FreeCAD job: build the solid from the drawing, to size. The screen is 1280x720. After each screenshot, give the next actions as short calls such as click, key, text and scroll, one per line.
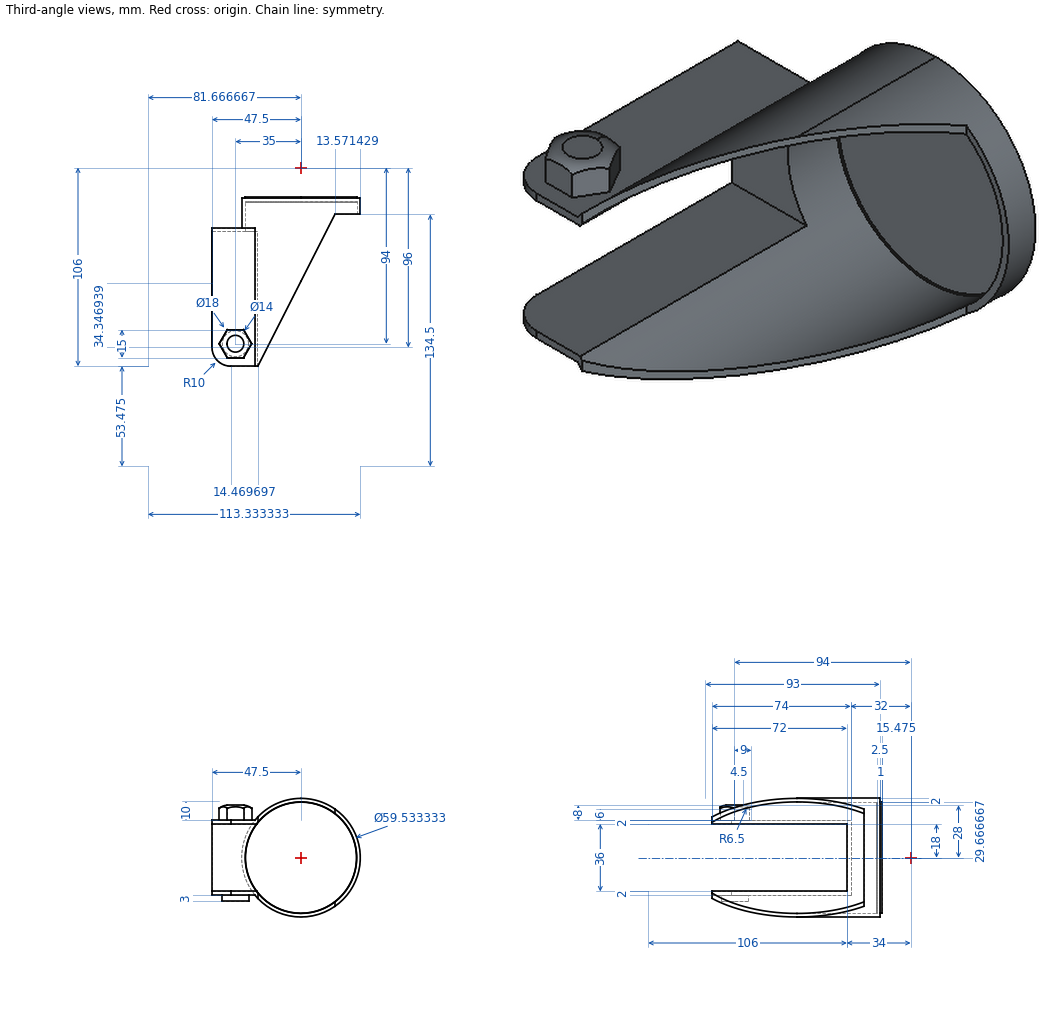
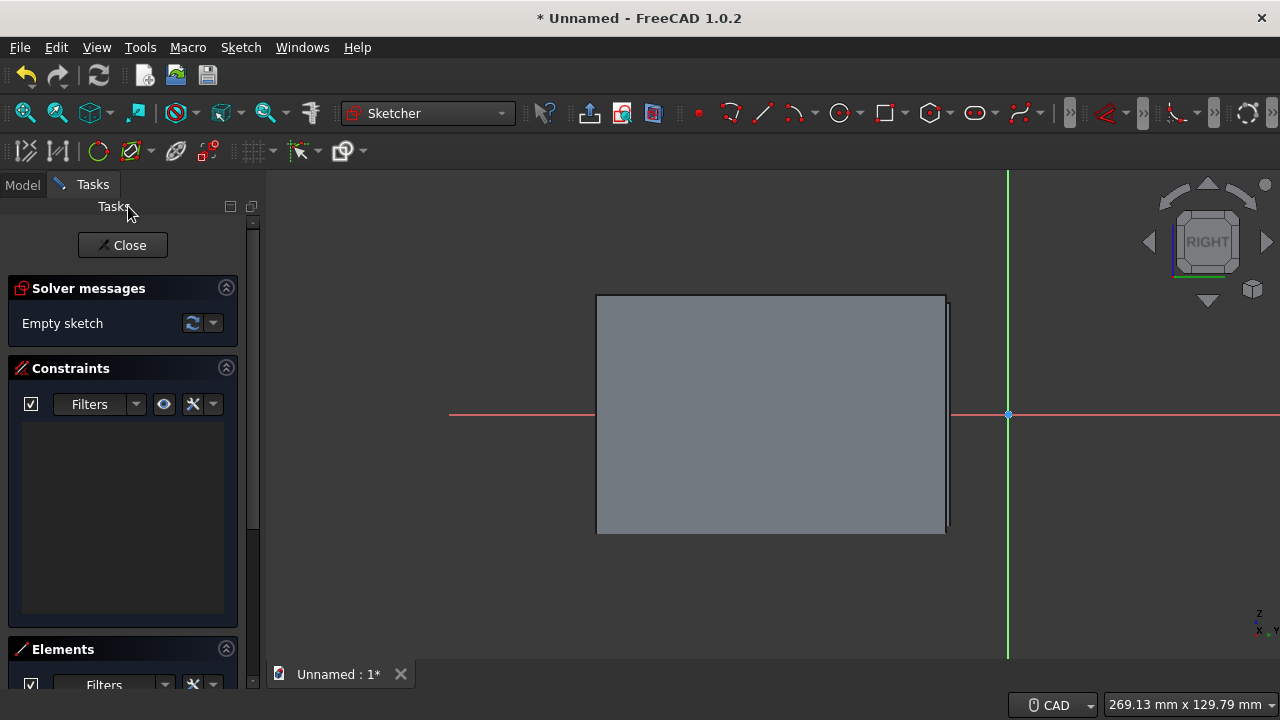
key(q)
key(s)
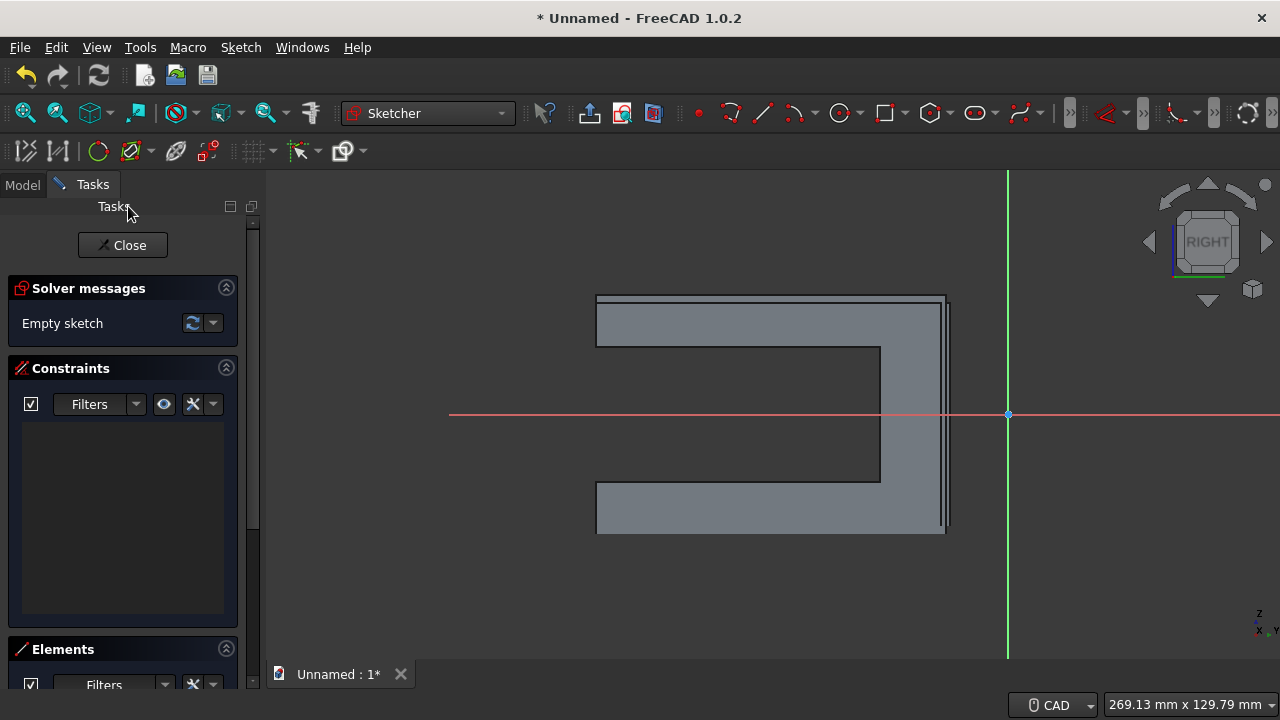
scroll(1021, 415, up, 2)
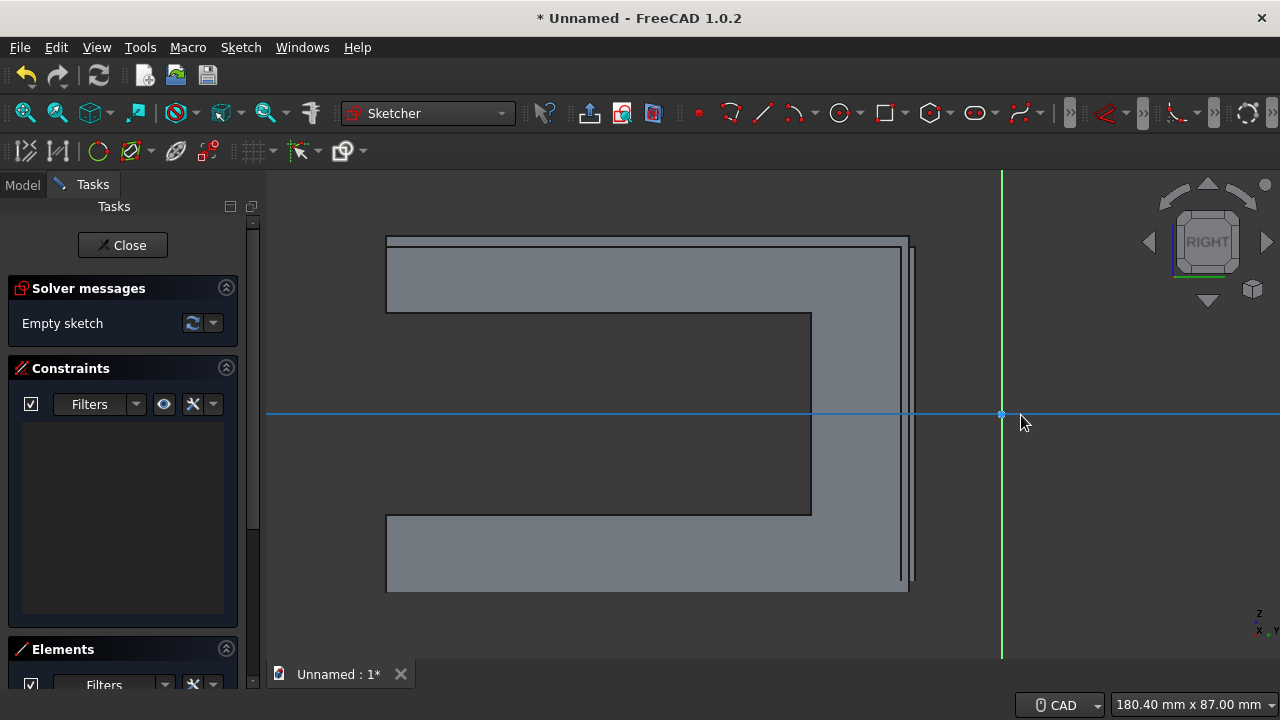
click(732, 114)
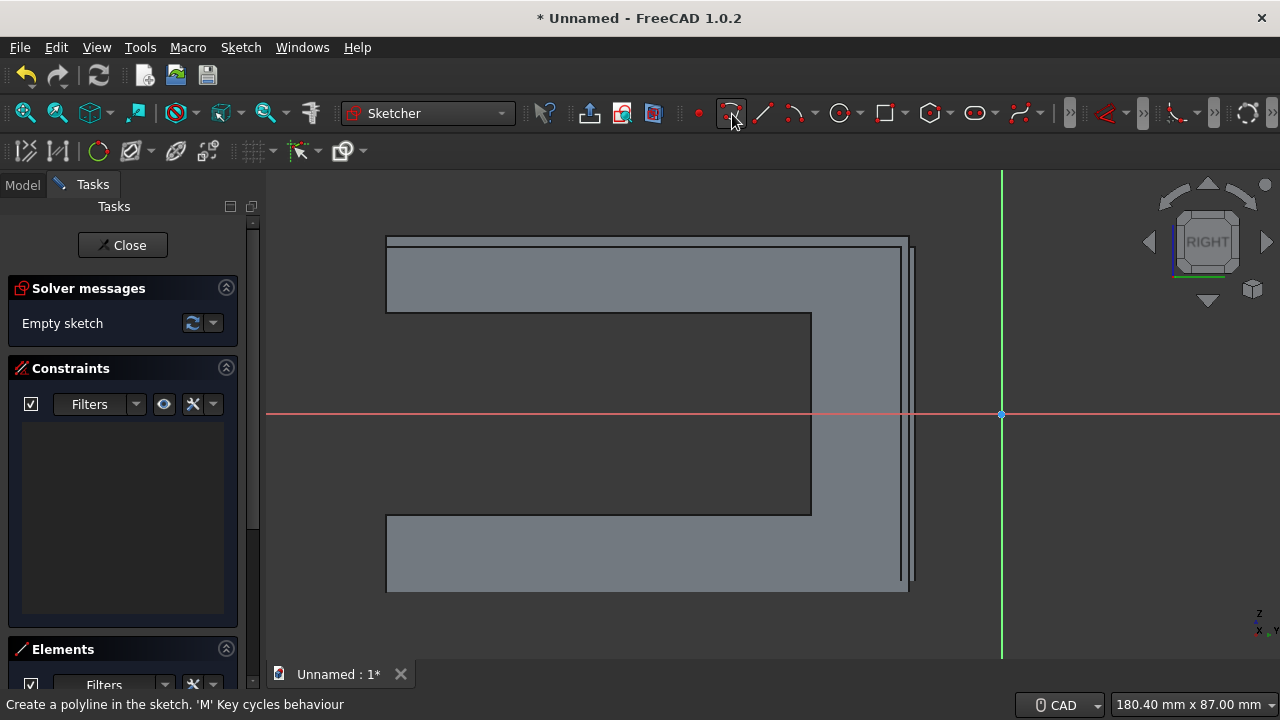
click(822, 302)
click(406, 302)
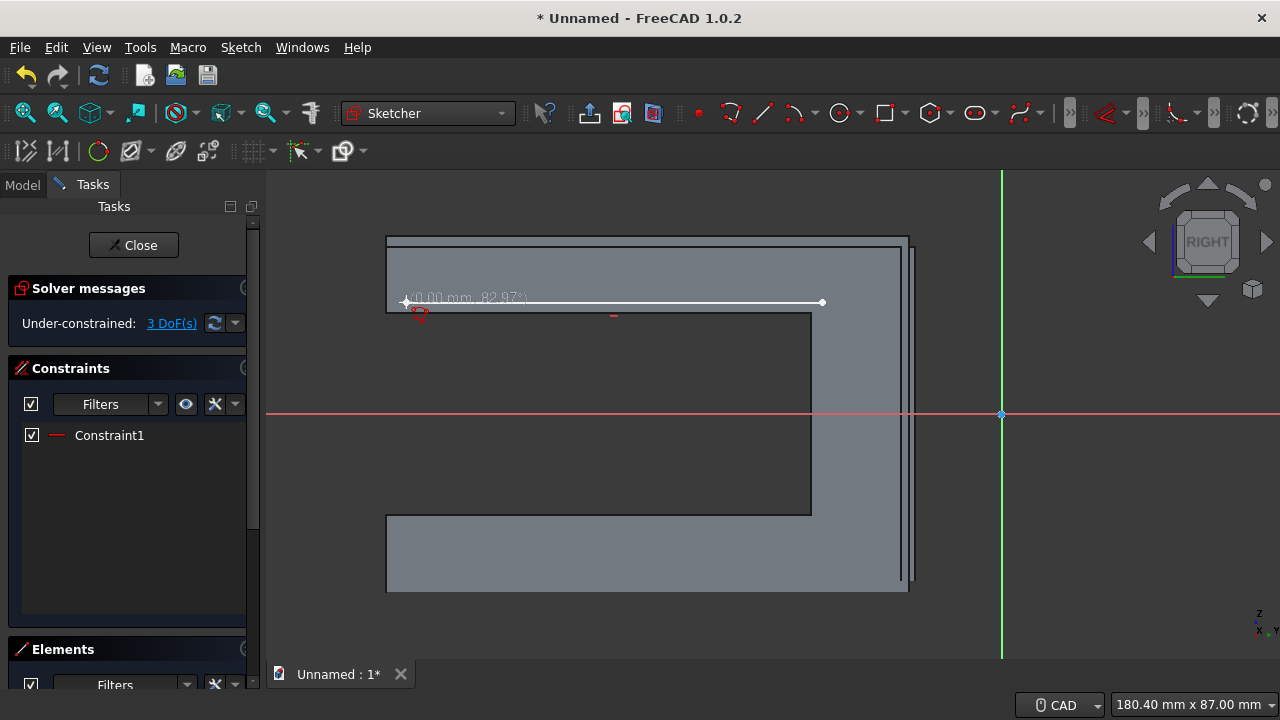
scroll(406, 313, up, 2)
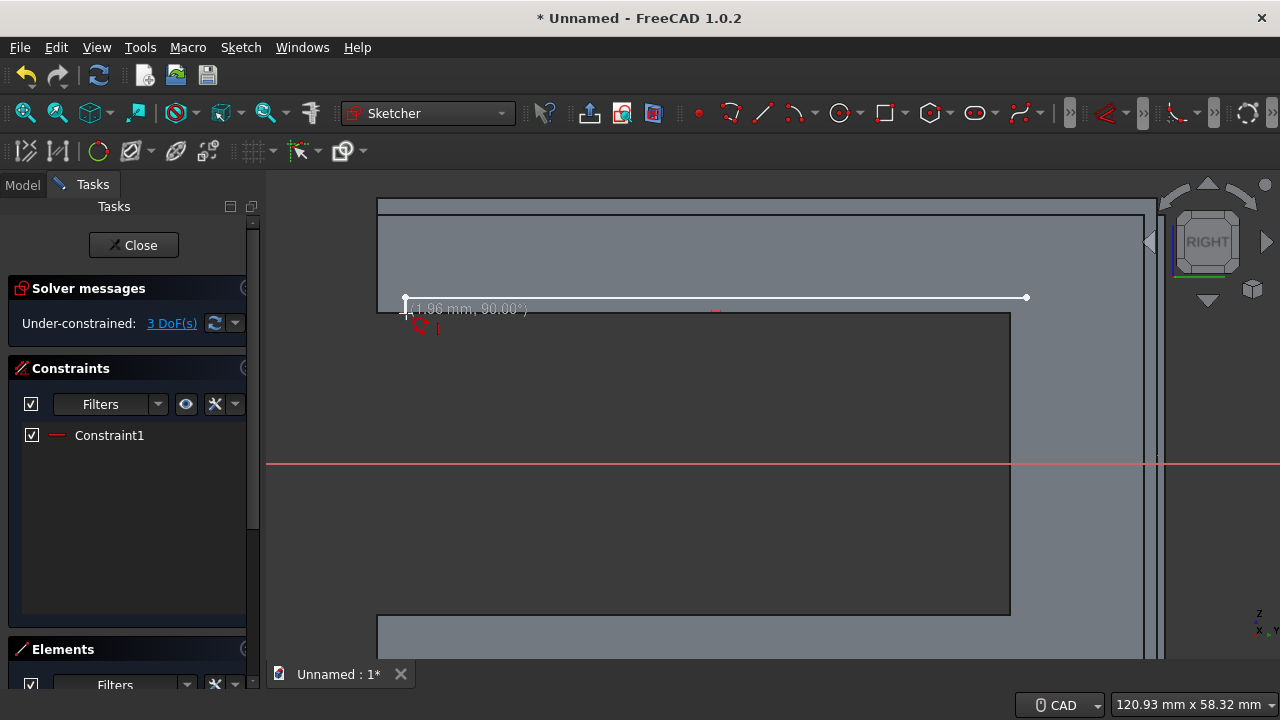
click(406, 313)
click(1010, 313)
click(1010, 615)
click(406, 615)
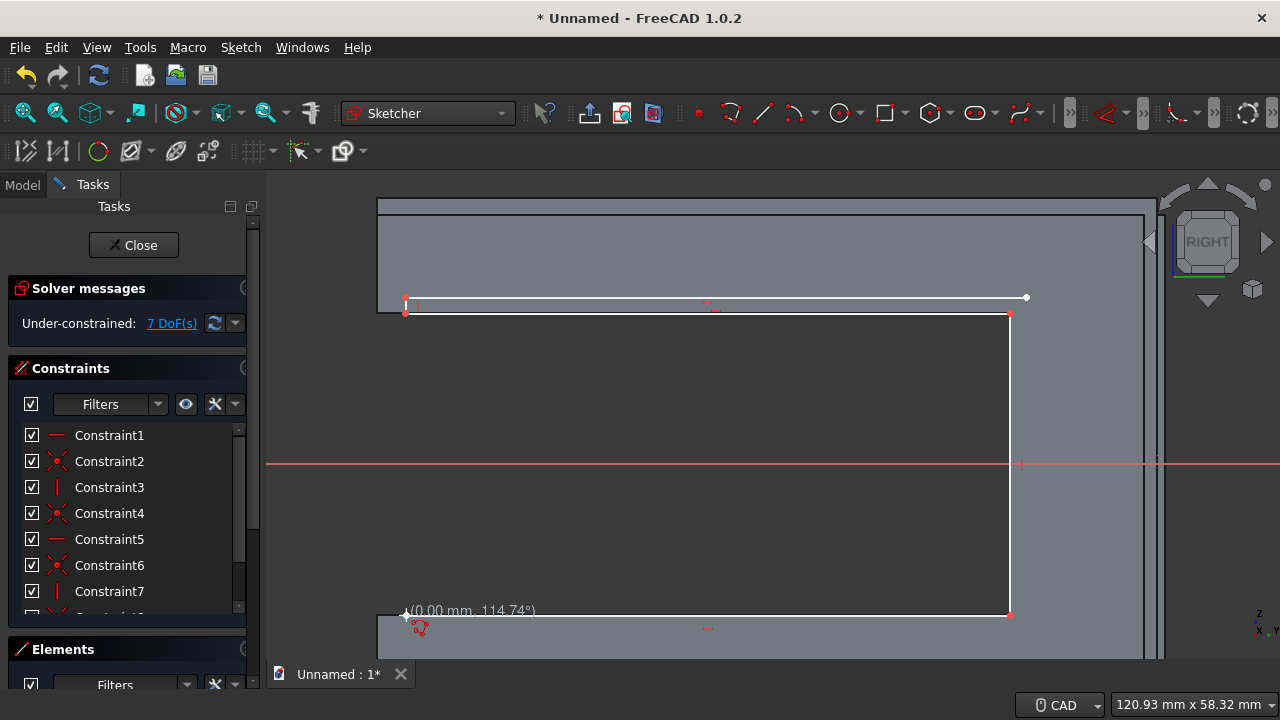
scroll(408, 314, down, 2)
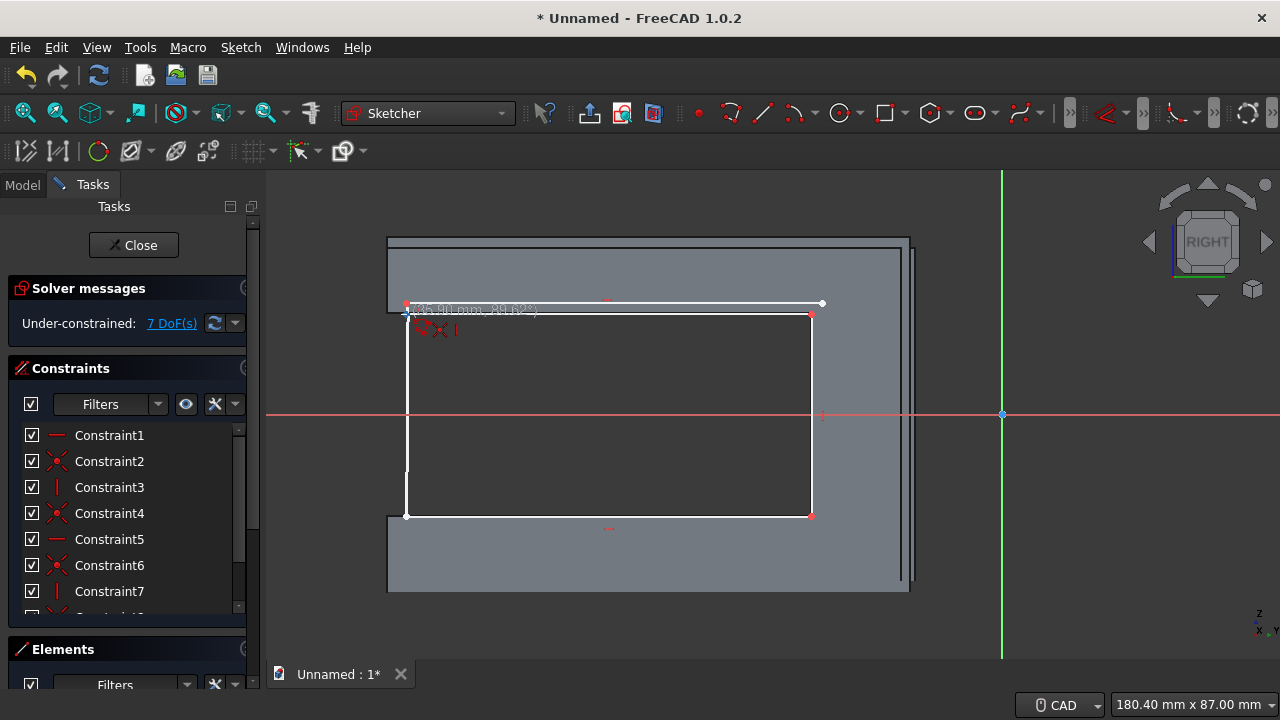
scroll(407, 527, up, 2)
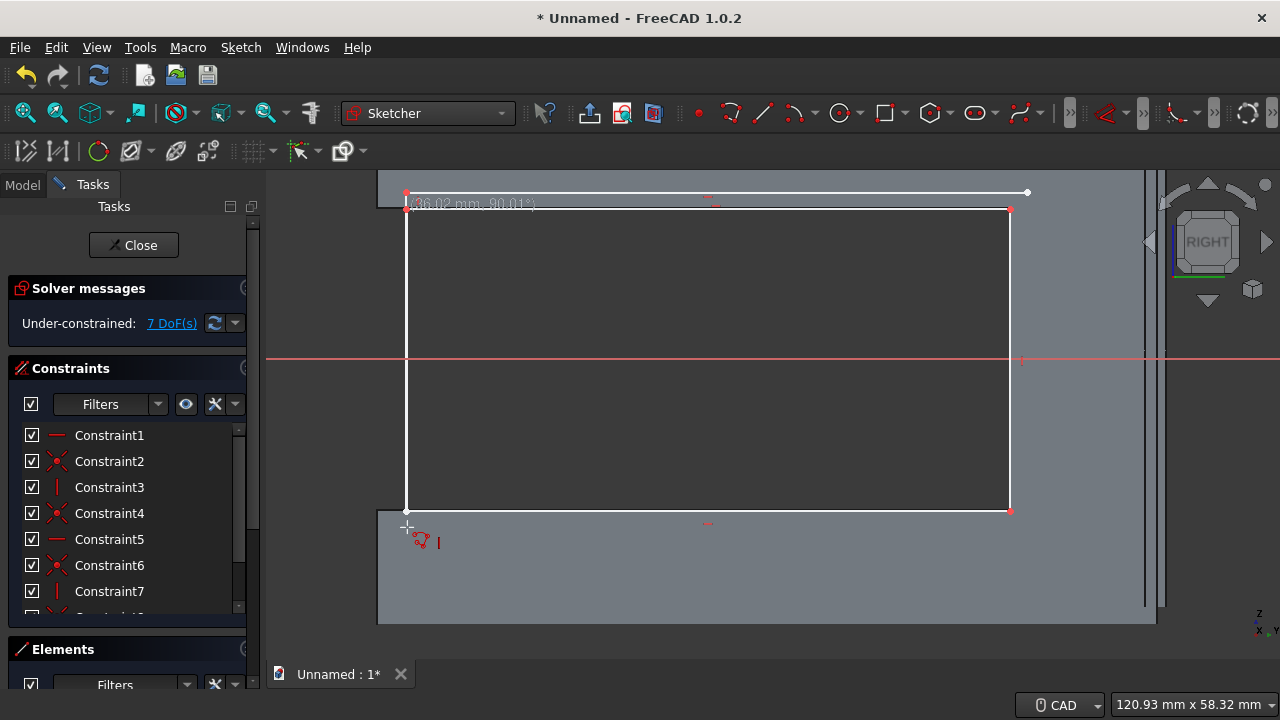
click(406, 527)
click(1027, 527)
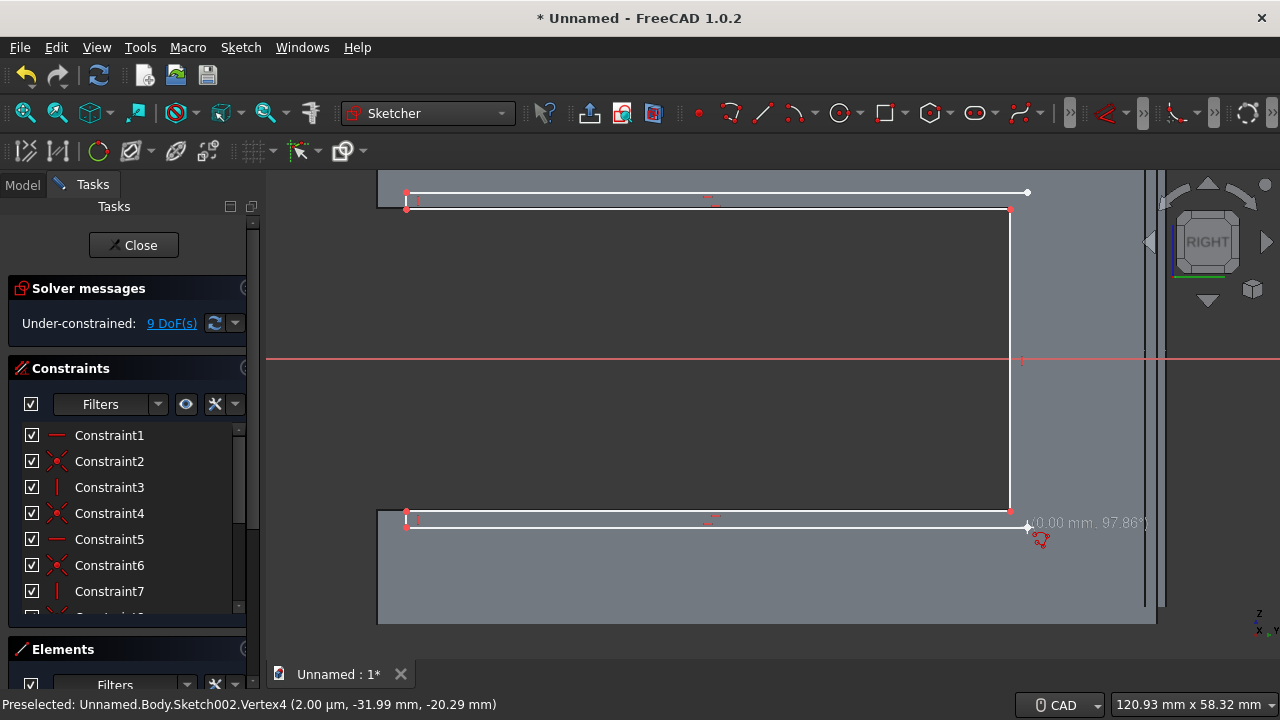
scroll(407, 528, down, 2)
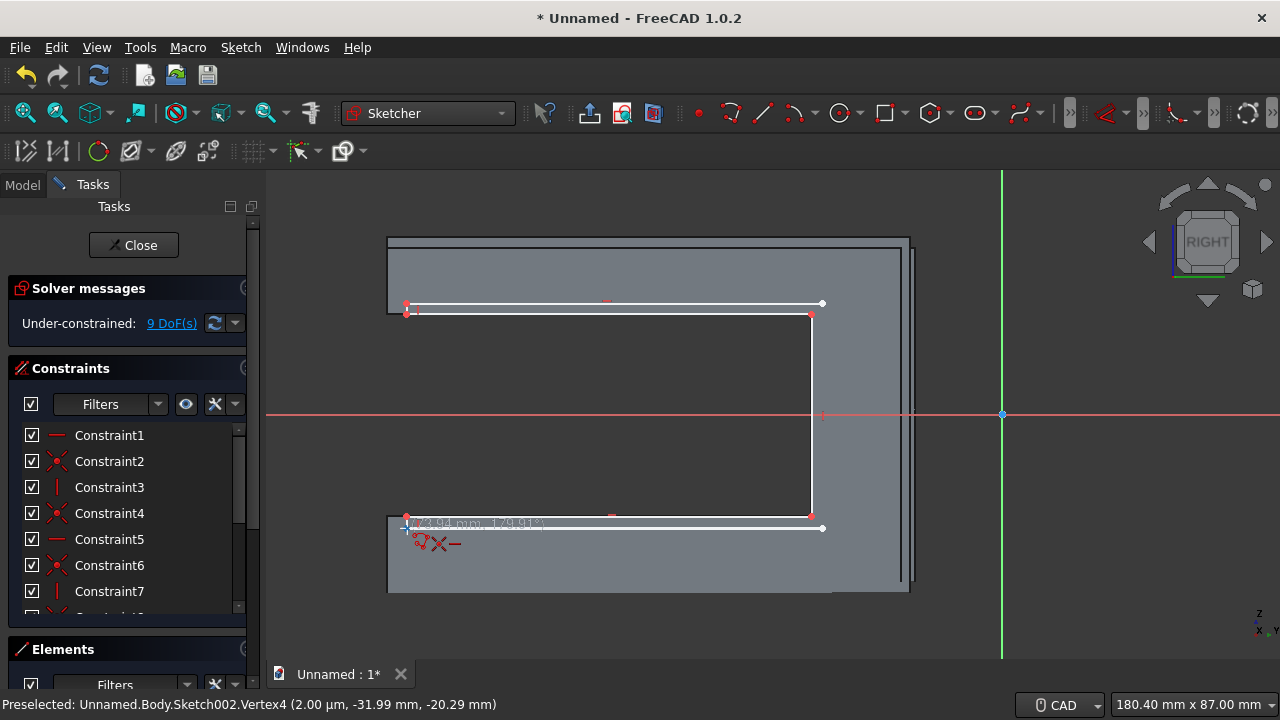
click(823, 304)
key(Escape)
key(Escape)